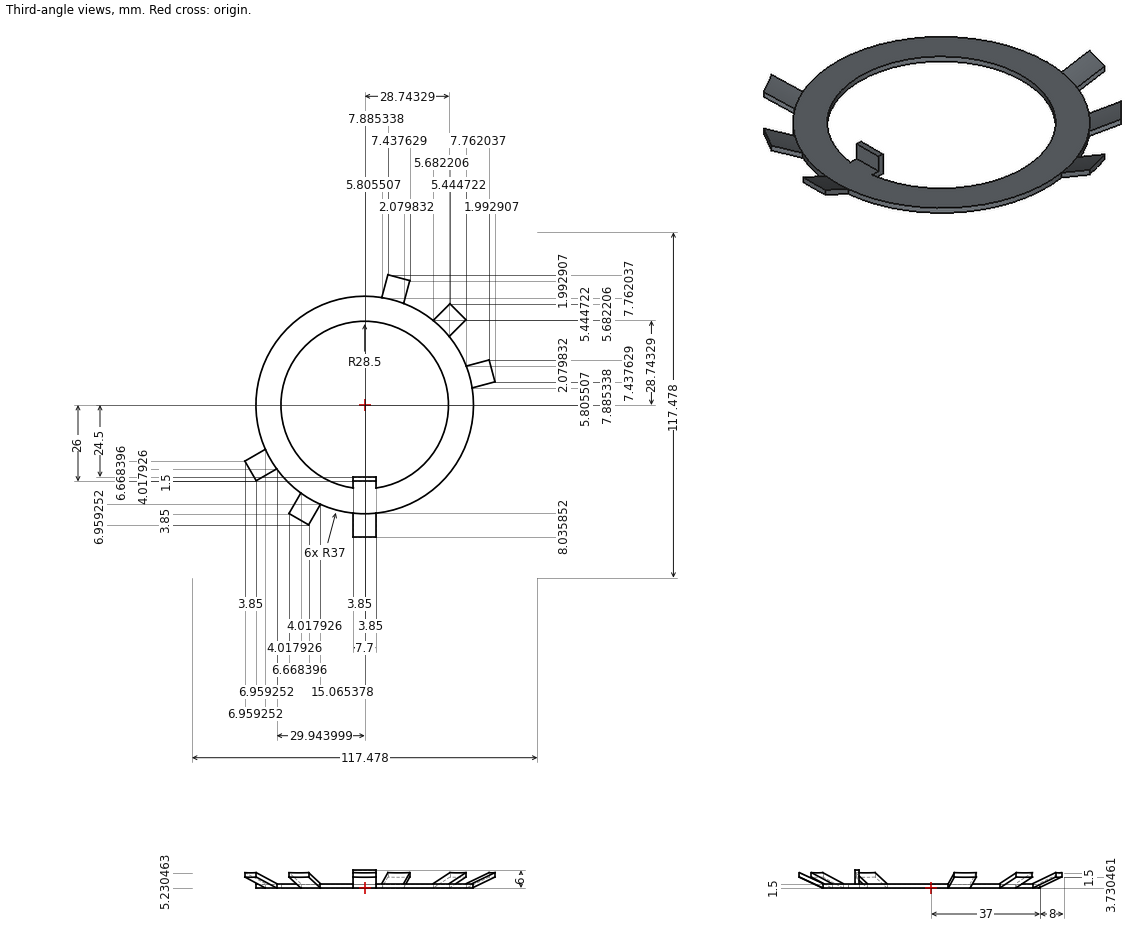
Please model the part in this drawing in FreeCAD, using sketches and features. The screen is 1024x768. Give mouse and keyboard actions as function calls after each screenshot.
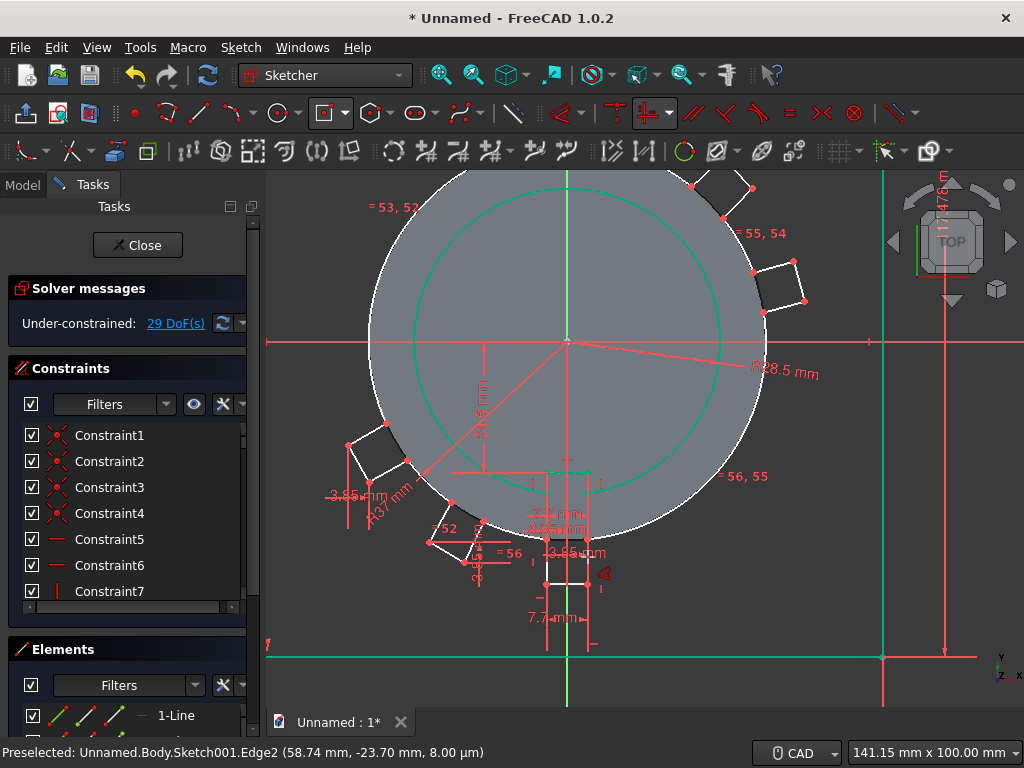
click(588, 557)
click(622, 577)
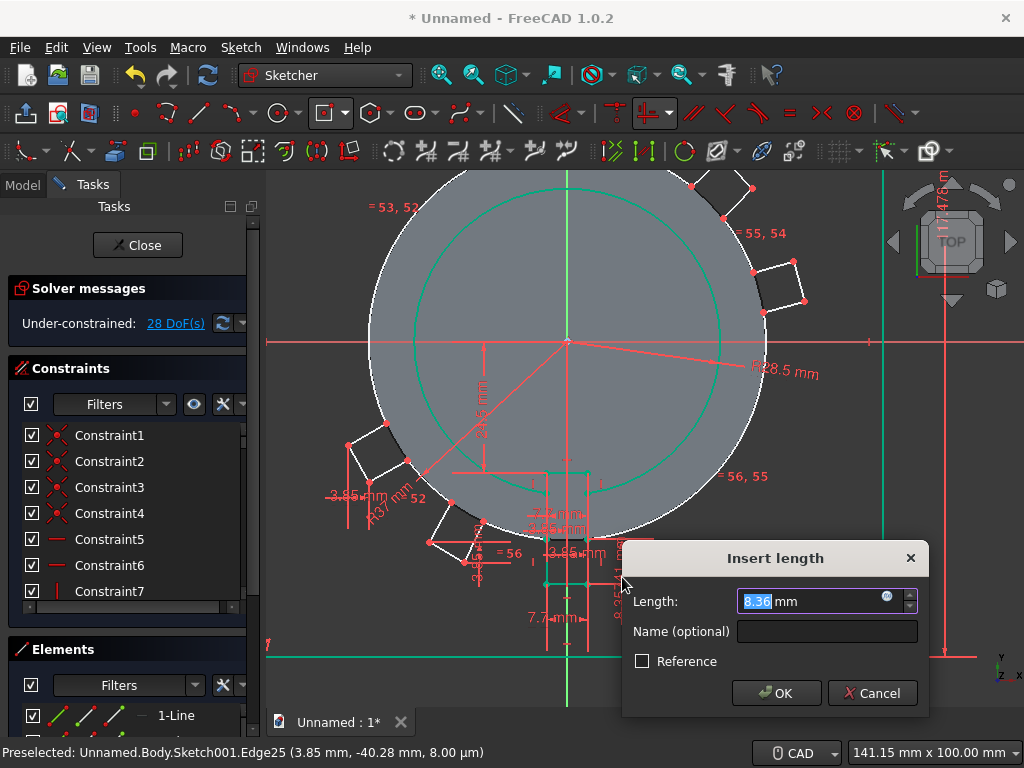
text(8.035852)
key(Return)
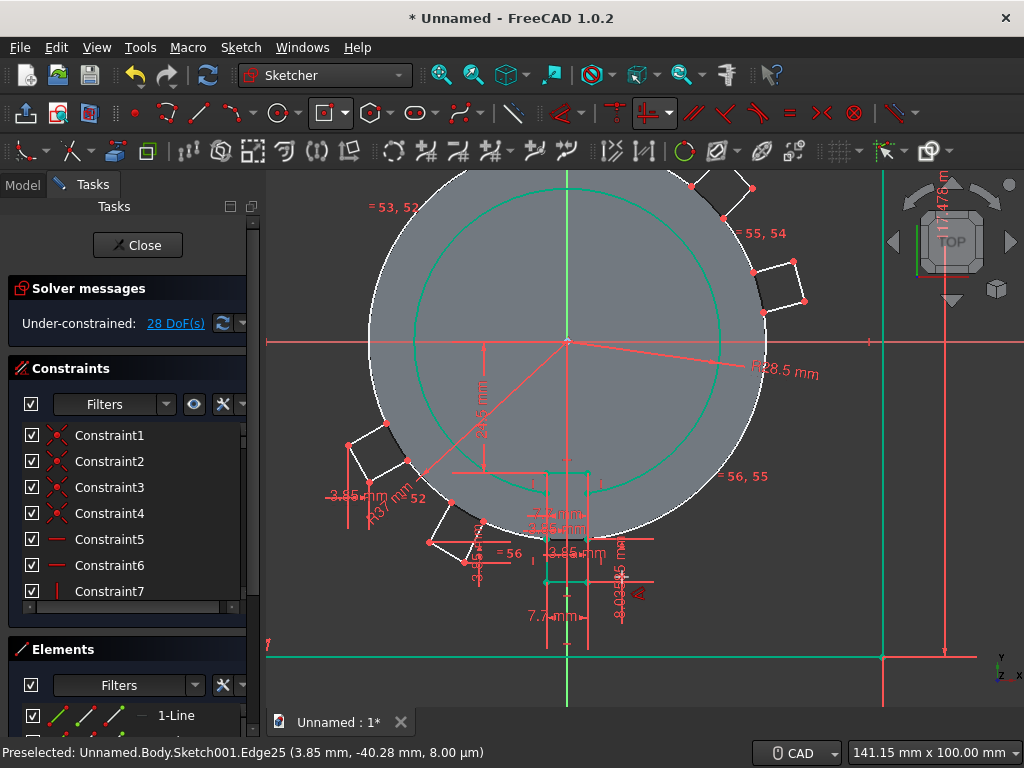
scroll(588, 556, down, 3)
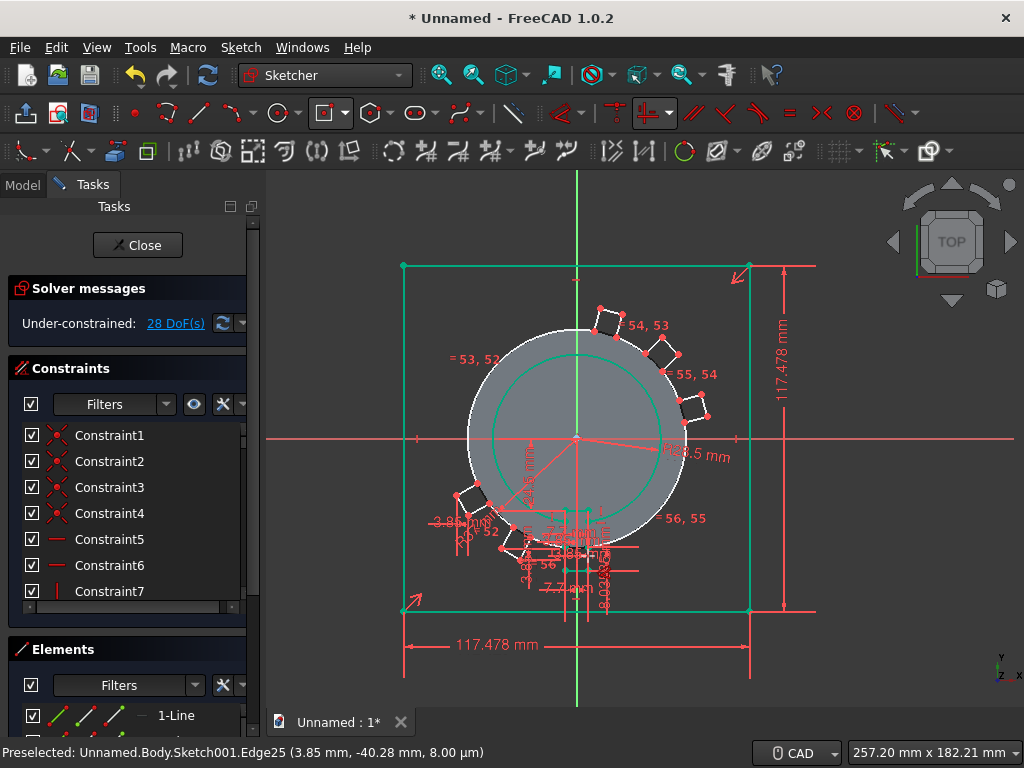
scroll(594, 331, up, 5)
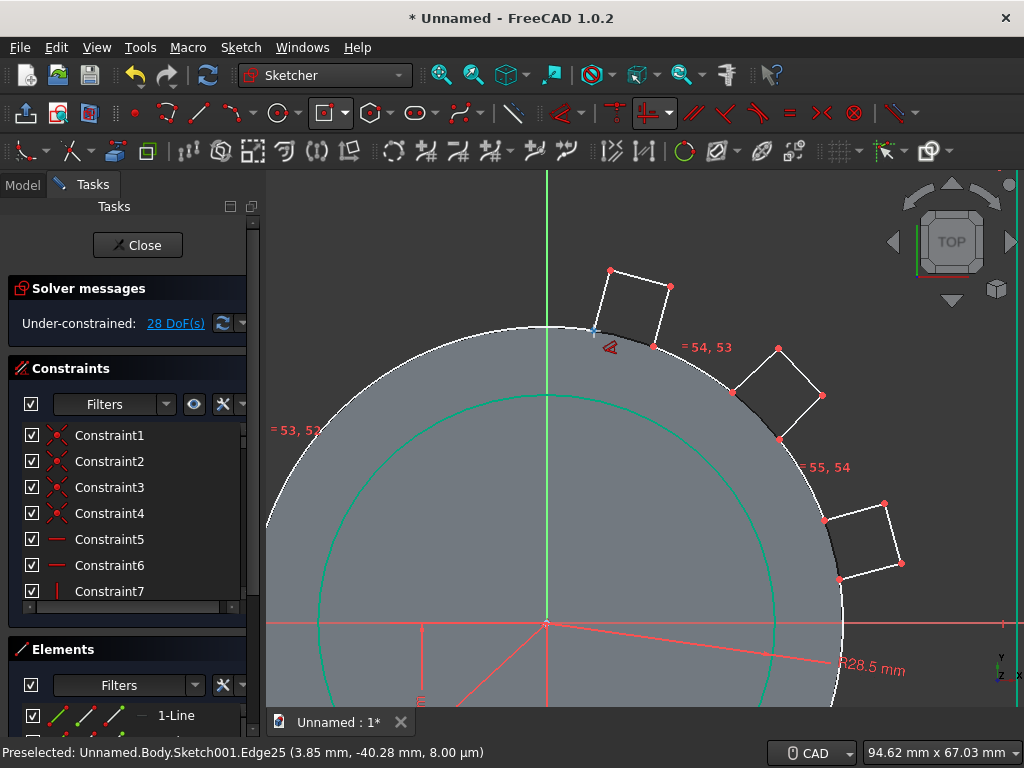
click(594, 331)
click(570, 297)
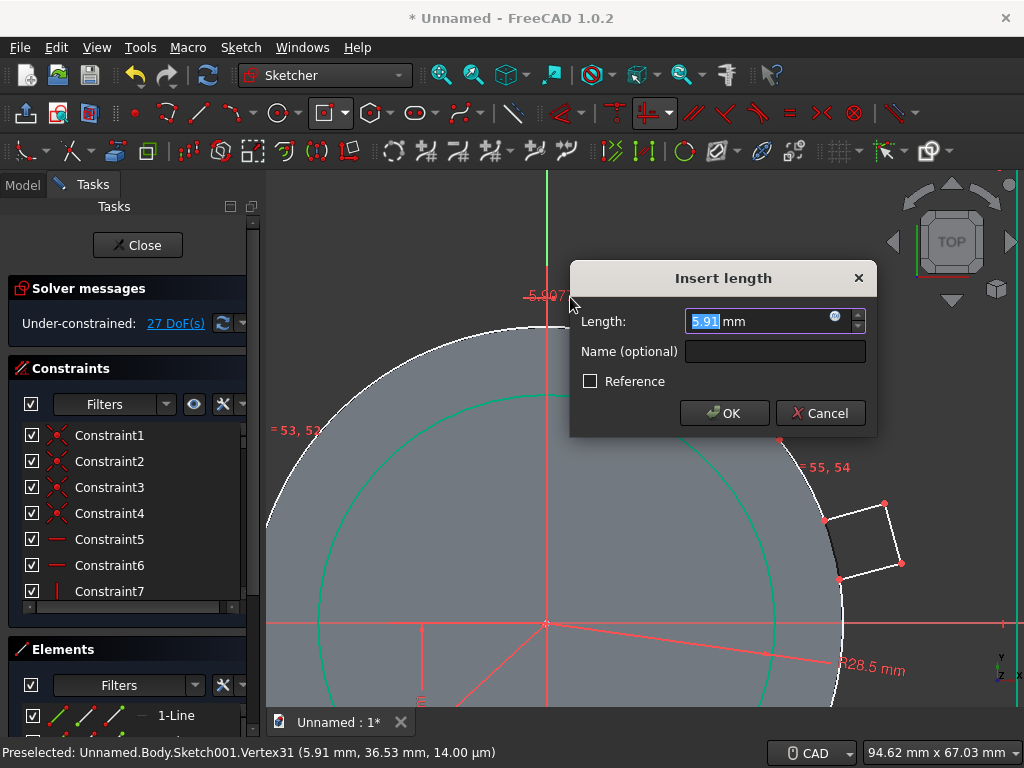
text(5.805507)
key(Return)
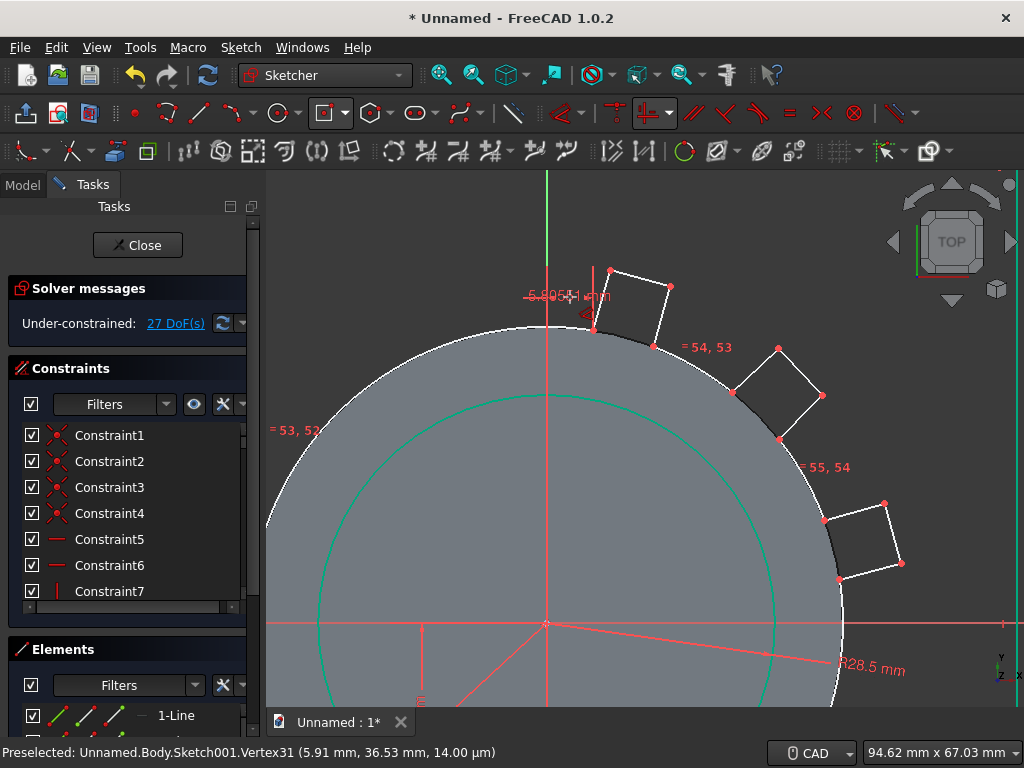
click(610, 270)
click(578, 236)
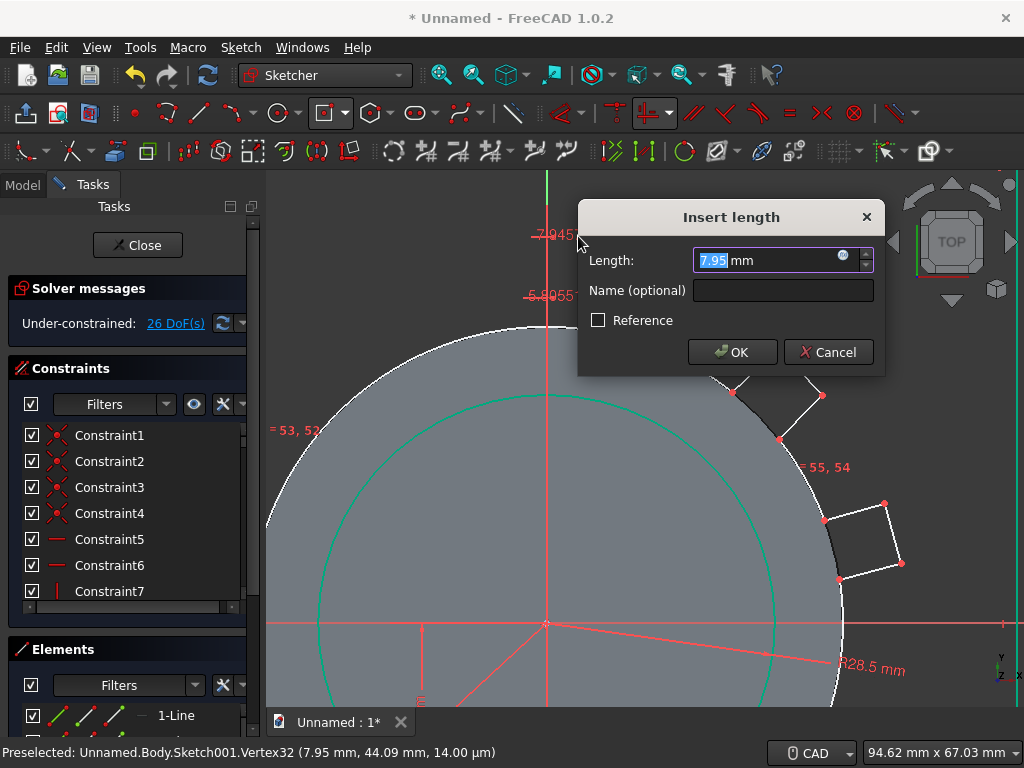
text(7.885338)
key(Return)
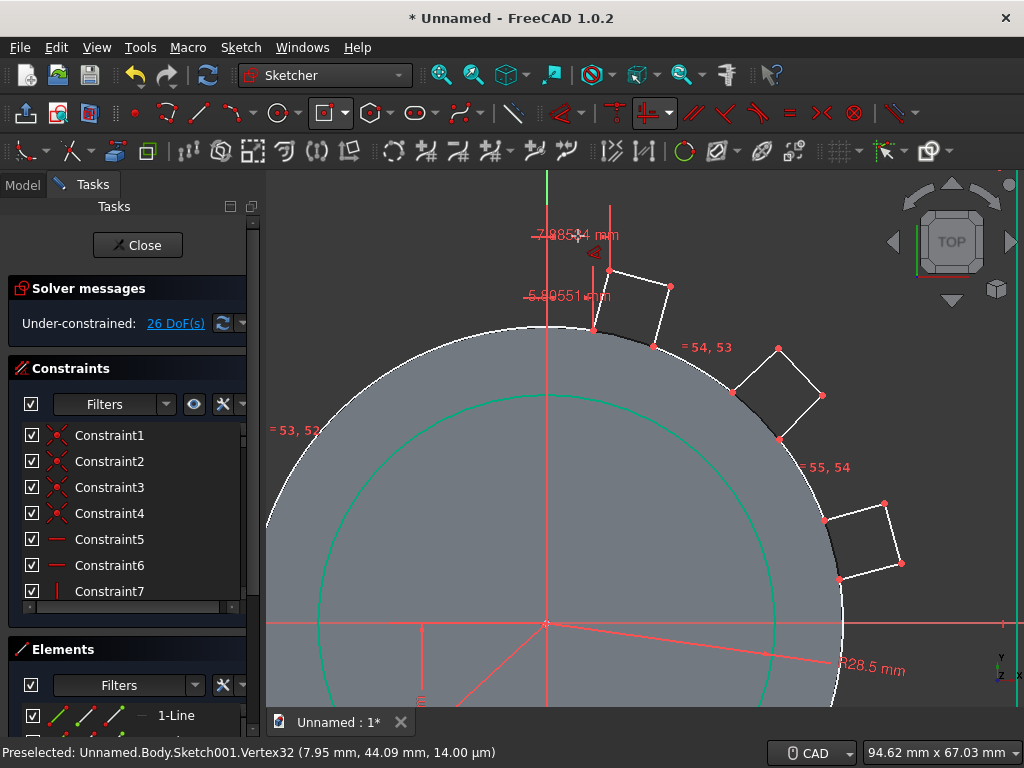
click(732, 392)
click(766, 508)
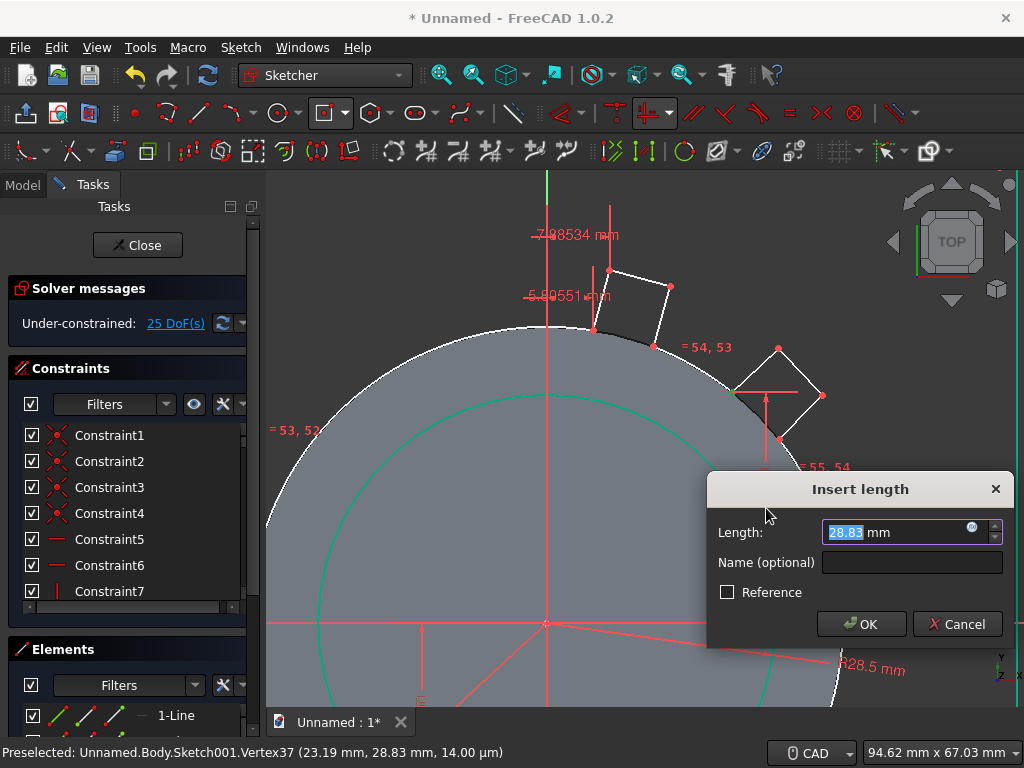
text(28.74329)
key(Return)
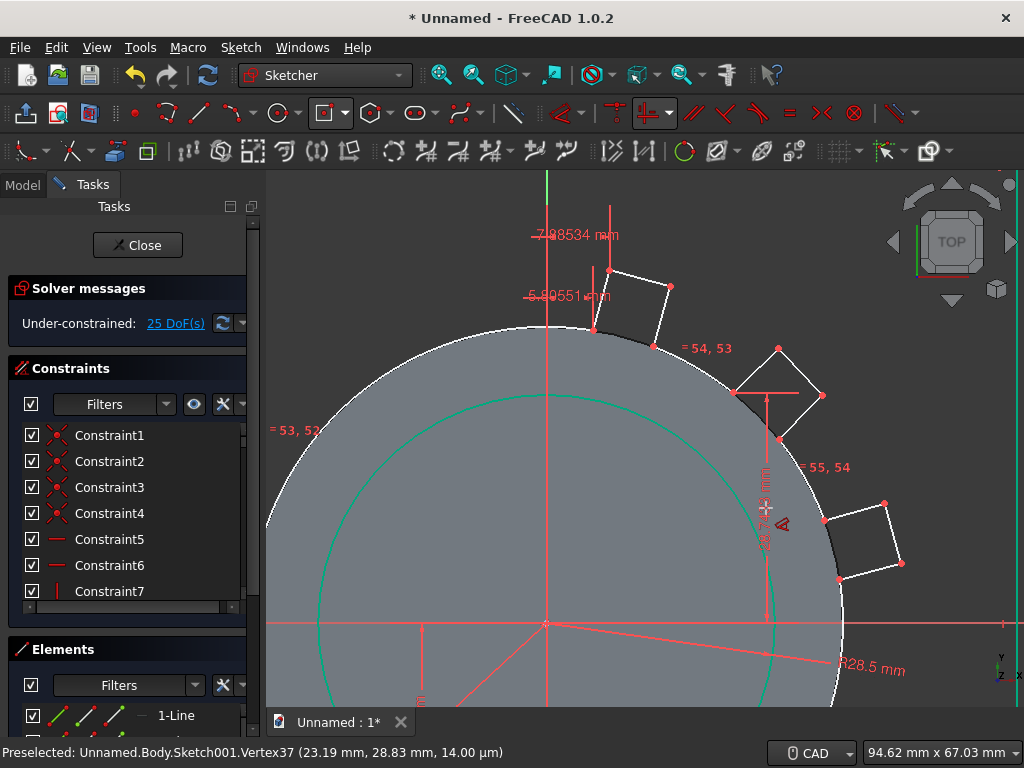
click(779, 439)
click(663, 405)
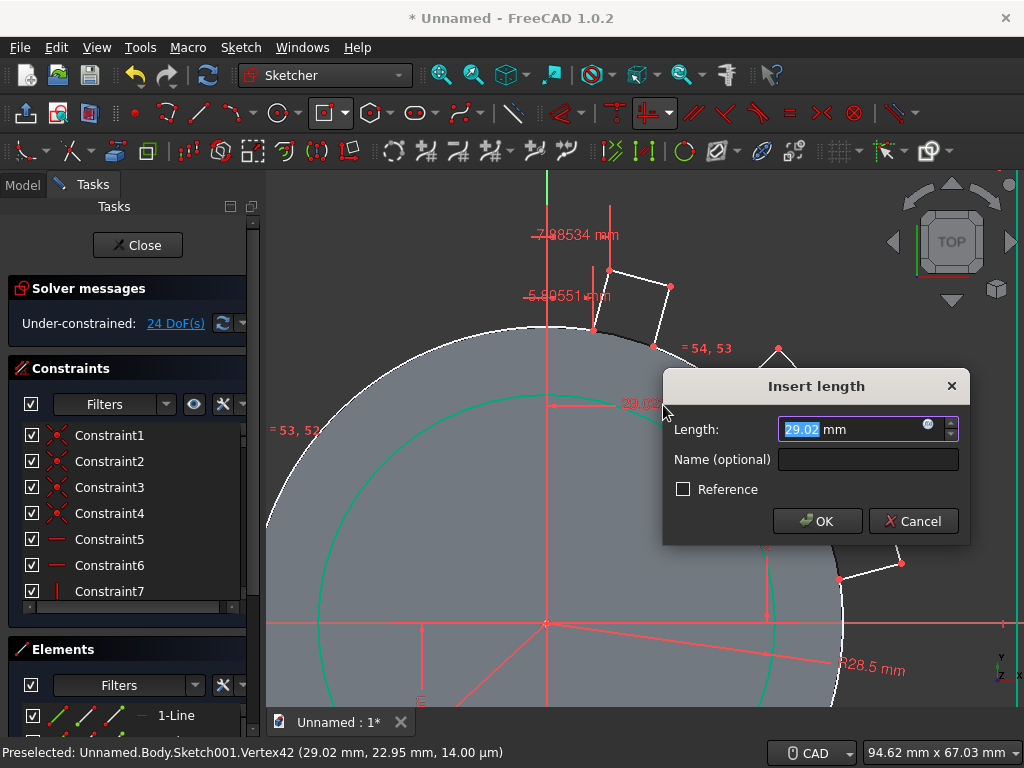
text(28.74329)
key(Return)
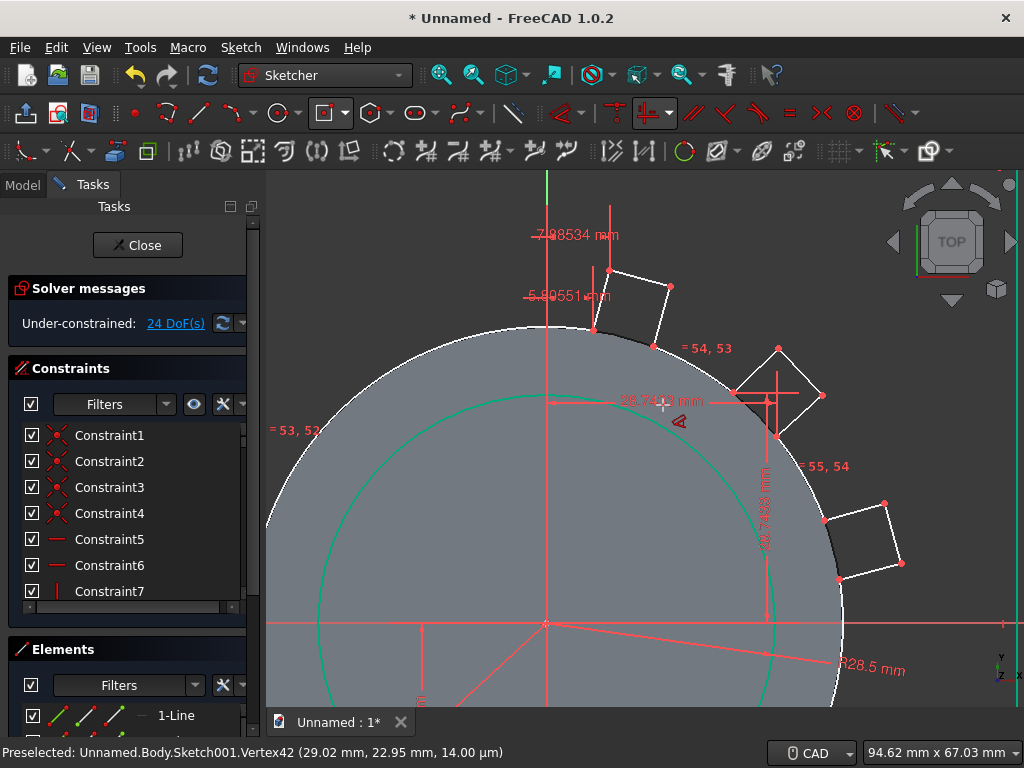
scroll(594, 331, down, 5)